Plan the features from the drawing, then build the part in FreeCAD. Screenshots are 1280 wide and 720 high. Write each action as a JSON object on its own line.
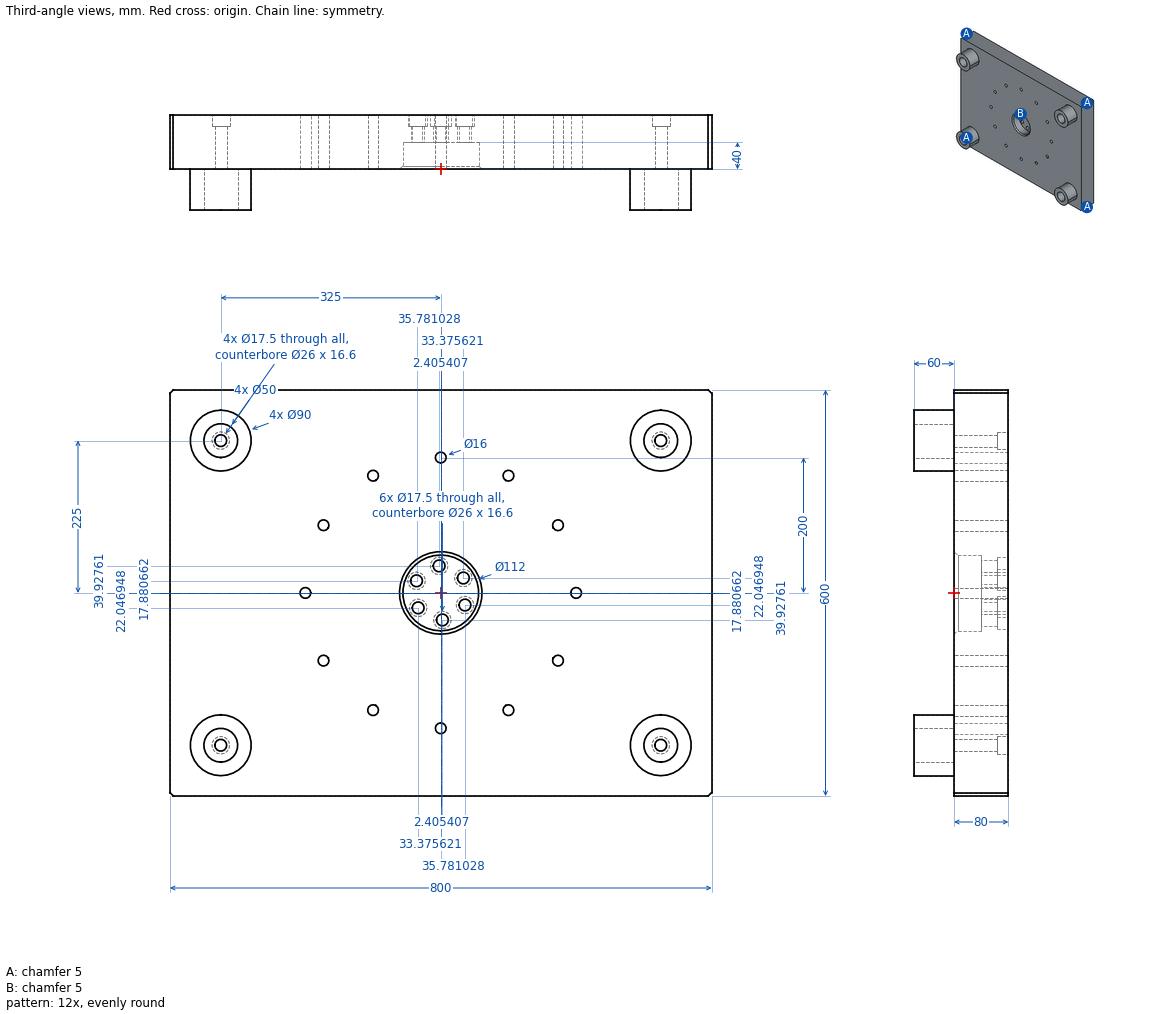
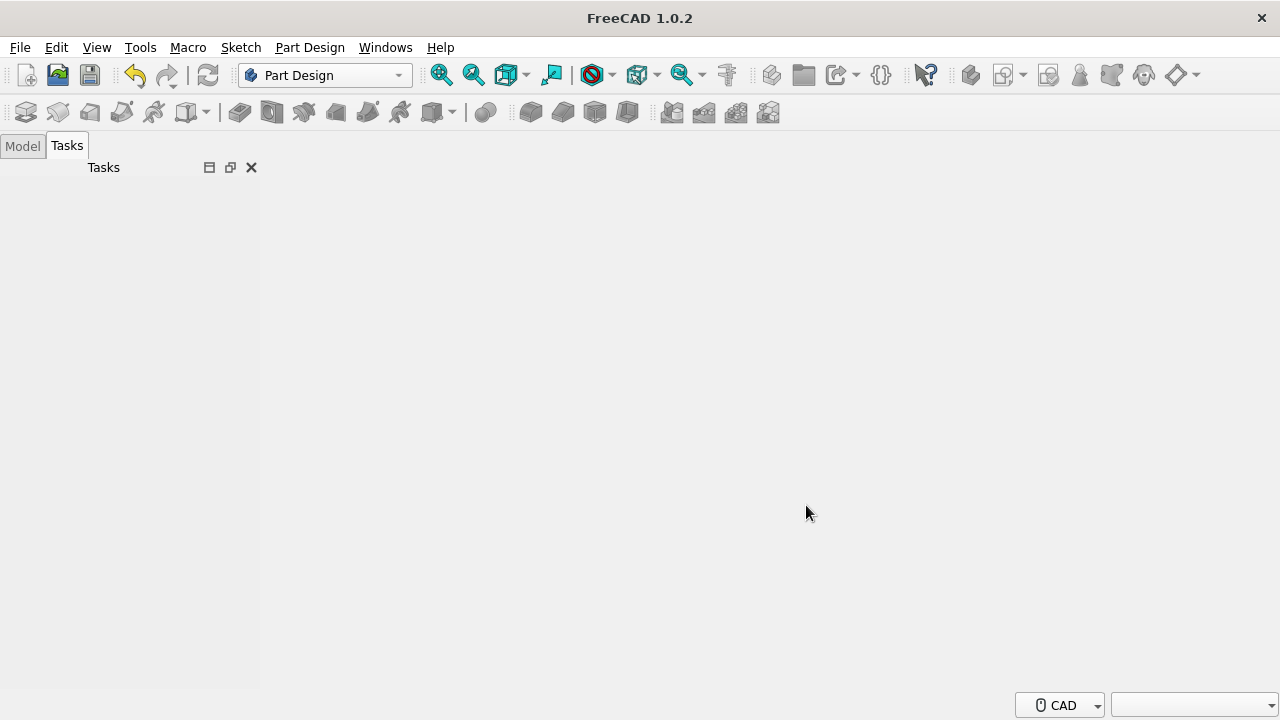
{"action": "key", "text": "ctrl+n"}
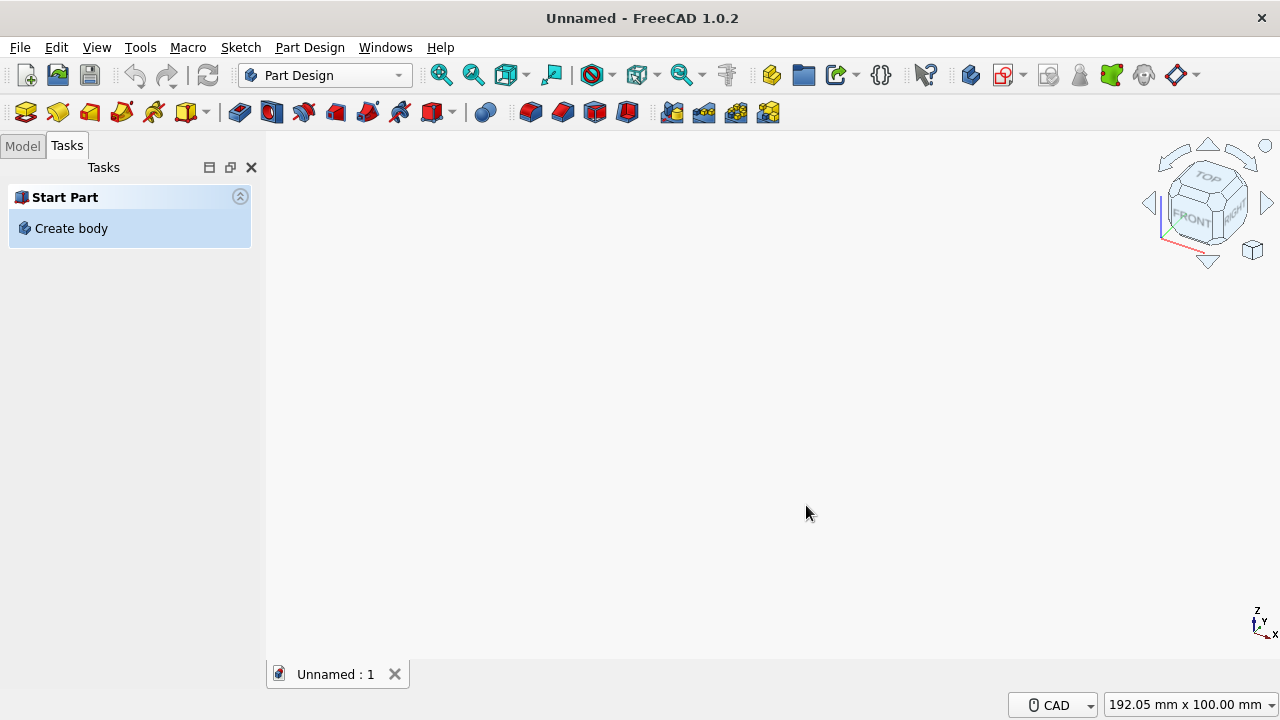
{"action": "left_click", "coordinate": [1004, 76]}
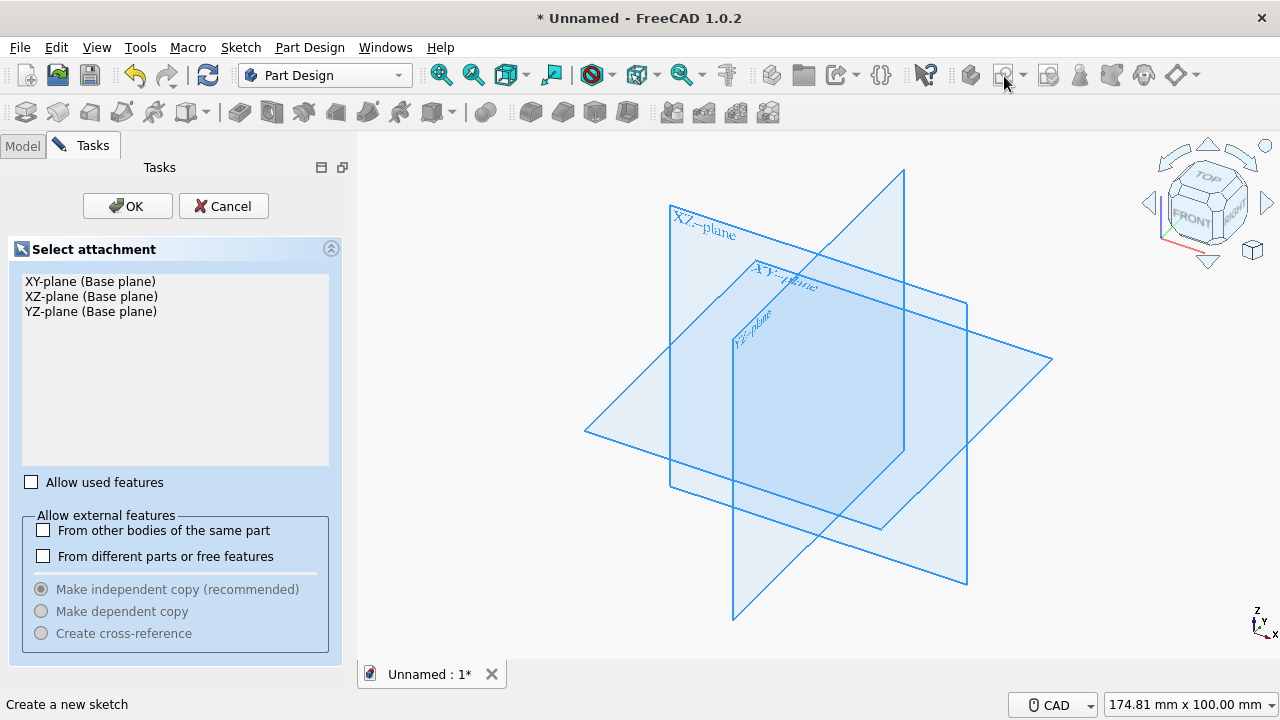
{"action": "left_click", "coordinate": [82, 296]}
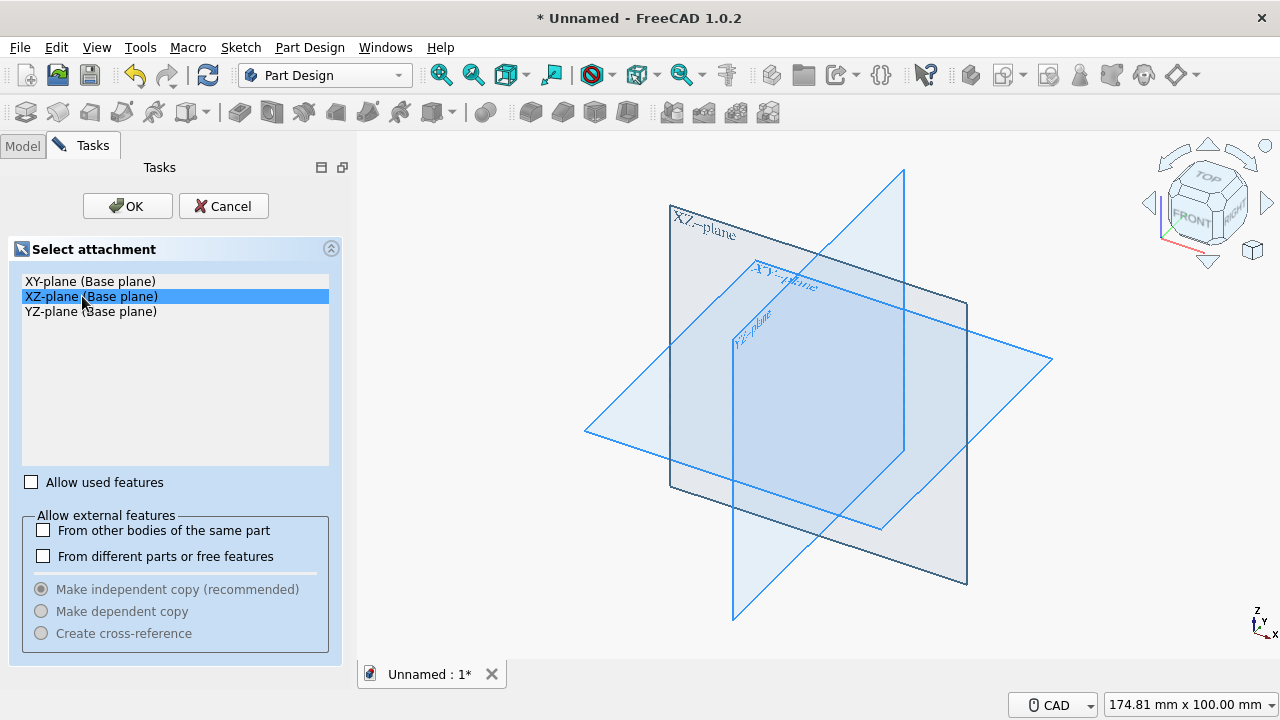
{"action": "left_click", "coordinate": [128, 206]}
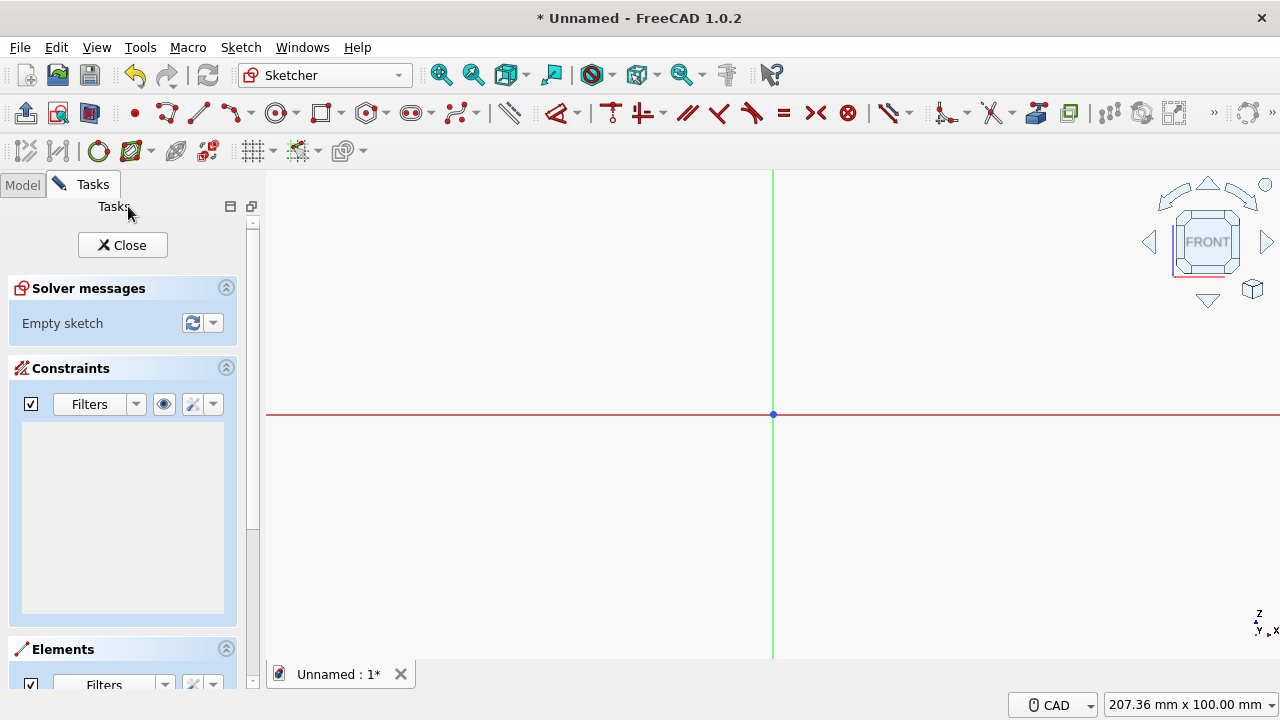
{"action": "scroll", "coordinate": [696, 414], "scroll_direction": "down", "scroll_amount": 11}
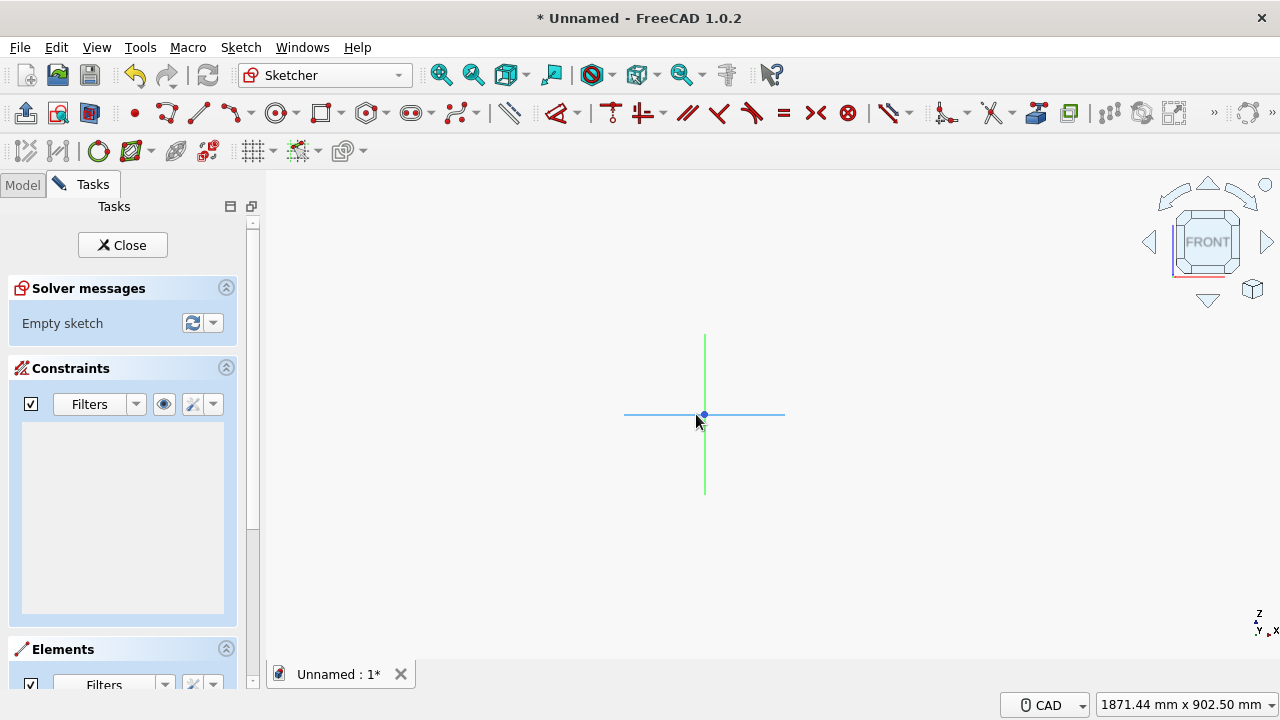
{"action": "left_click", "coordinate": [344, 114]}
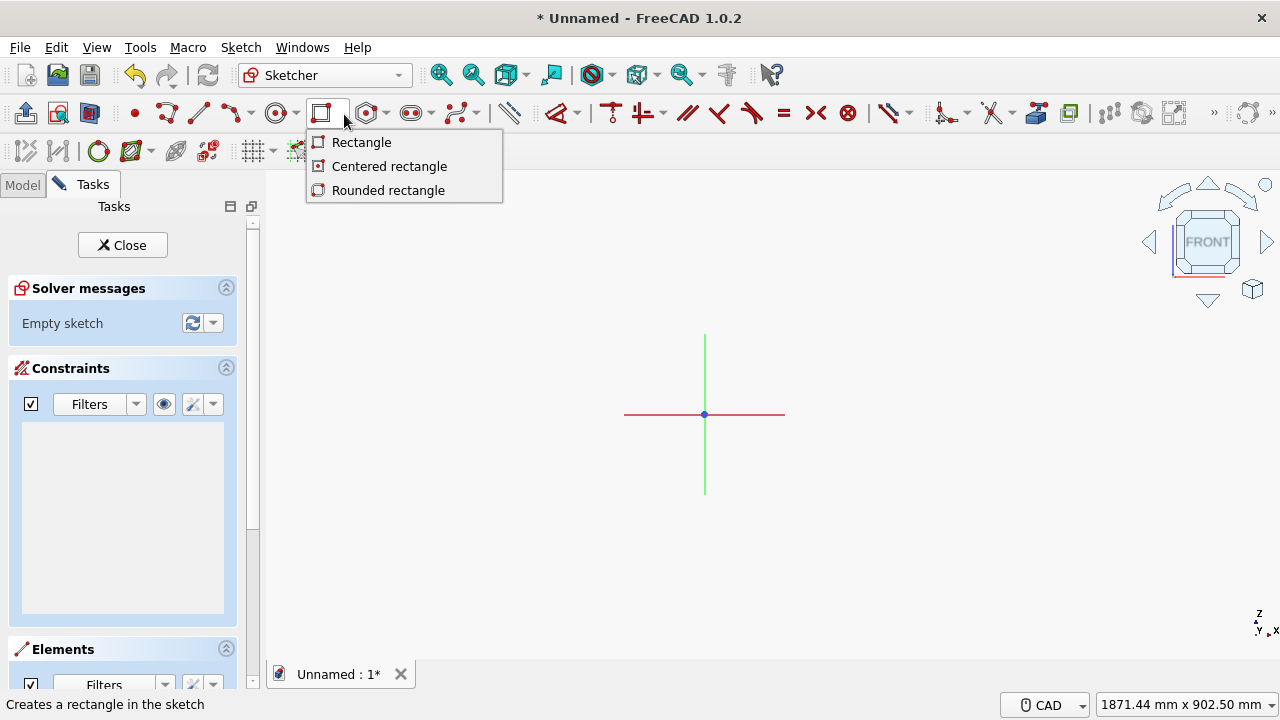
{"action": "left_click", "coordinate": [404, 166]}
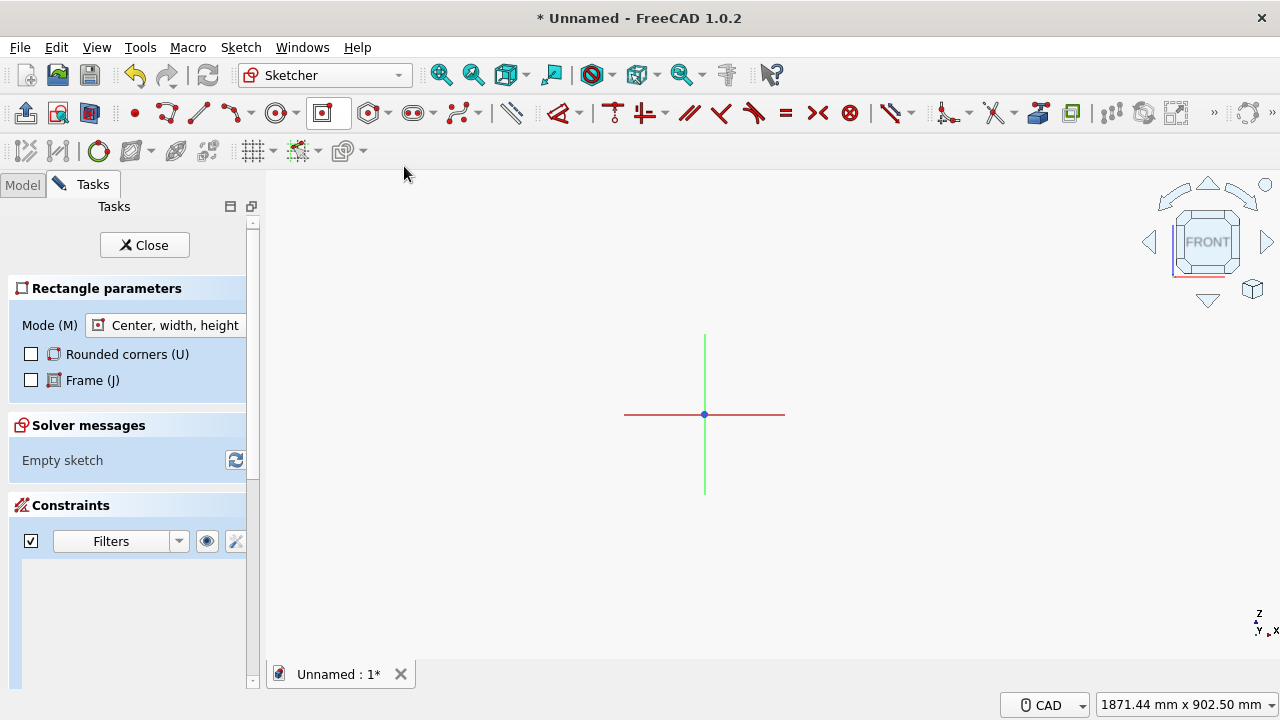
{"action": "left_click", "coordinate": [705, 414]}
{"action": "mouse_move", "coordinate": [922, 252]}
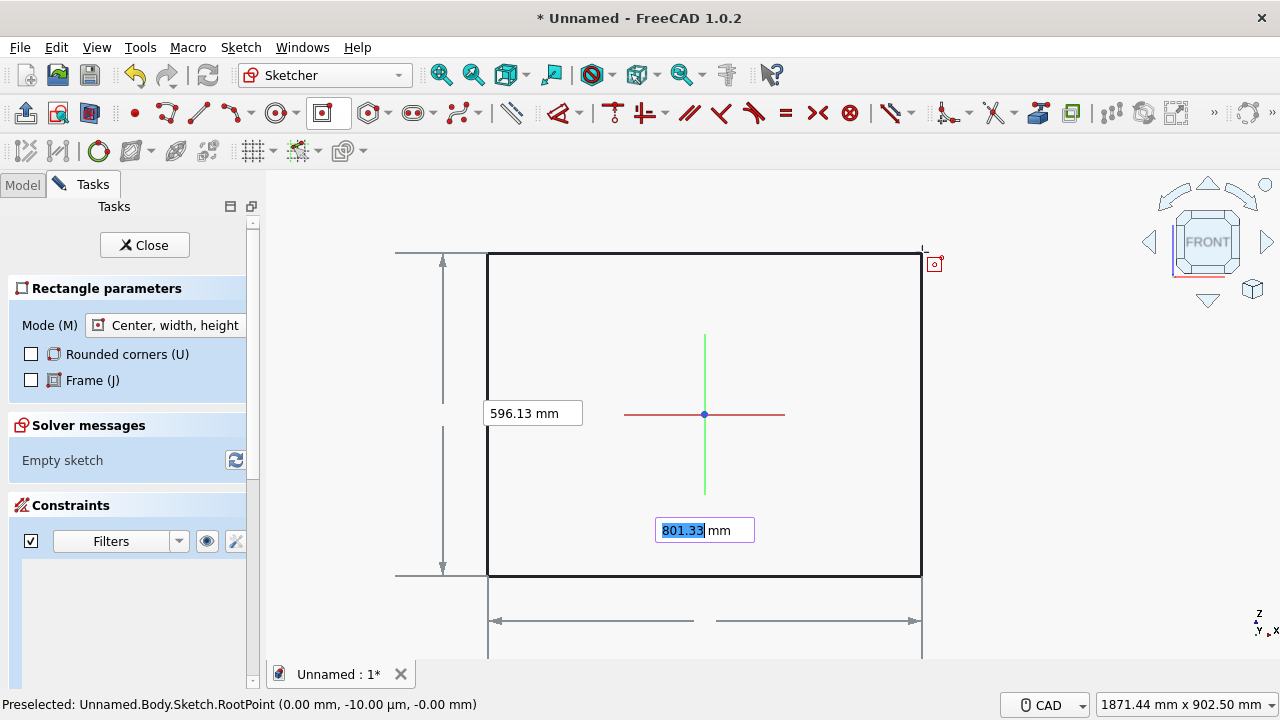
{"action": "type", "text": "800"}
{"action": "key", "text": "Tab"}
{"action": "type", "text": "600"}
{"action": "key", "text": "Return"}
{"action": "key", "text": "Escape"}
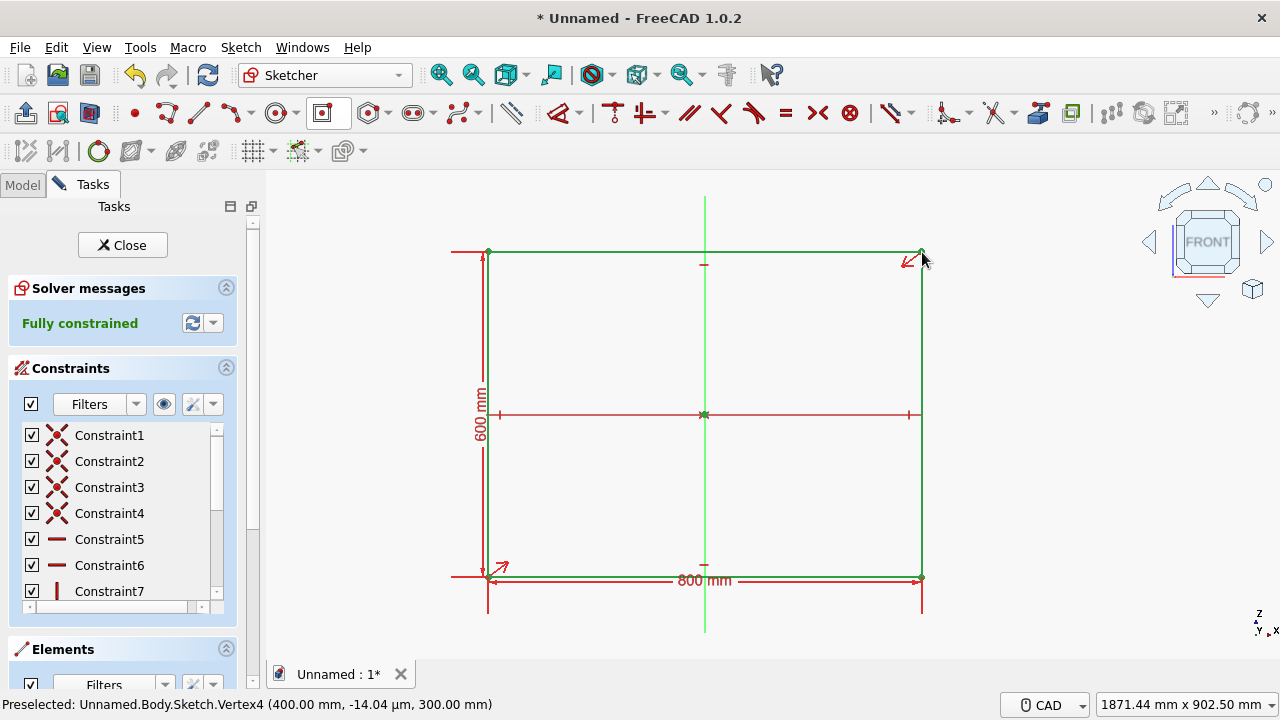
{"action": "left_click", "coordinate": [123, 245]}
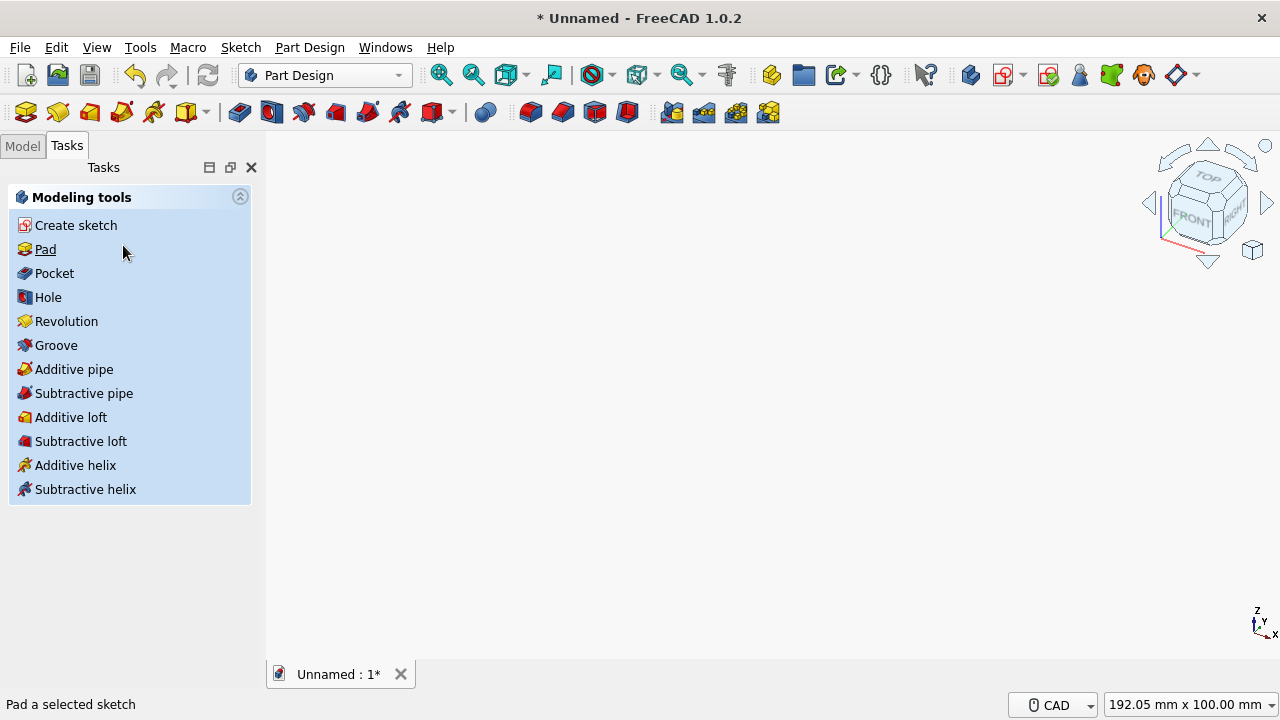
{"action": "left_click", "coordinate": [26, 112]}